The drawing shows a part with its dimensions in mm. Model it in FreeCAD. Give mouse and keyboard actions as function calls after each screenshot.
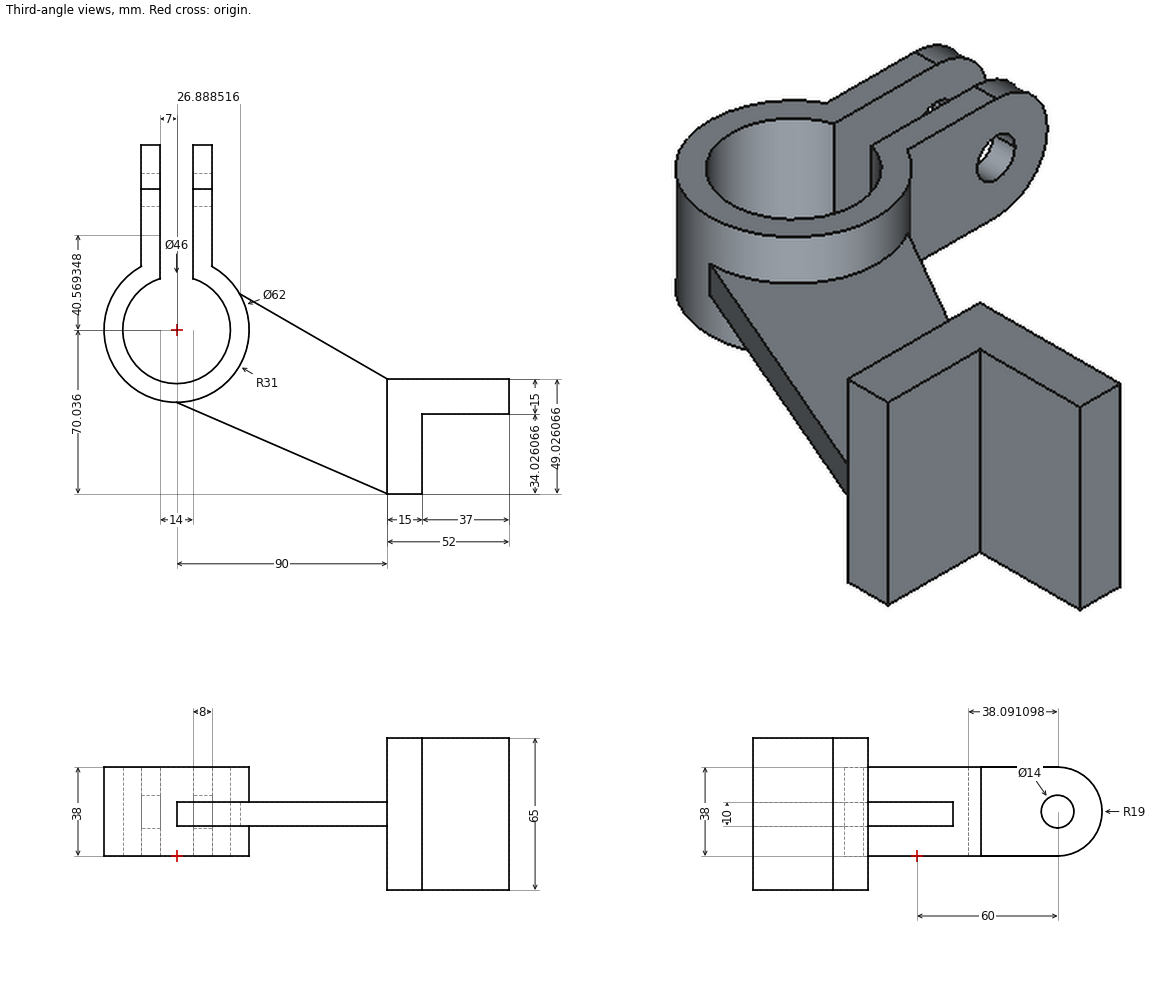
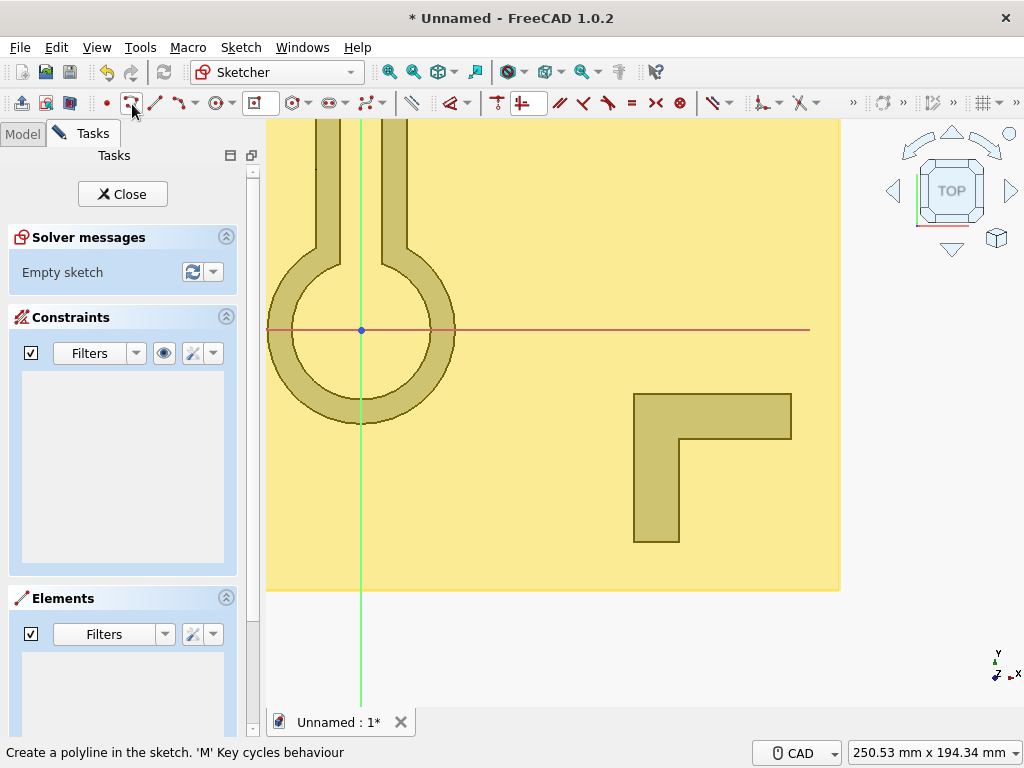
click(361, 424)
click(634, 542)
click(679, 542)
click(679, 439)
click(791, 439)
click(791, 394)
click(634, 394)
click(443, 283)
right_click(443, 283)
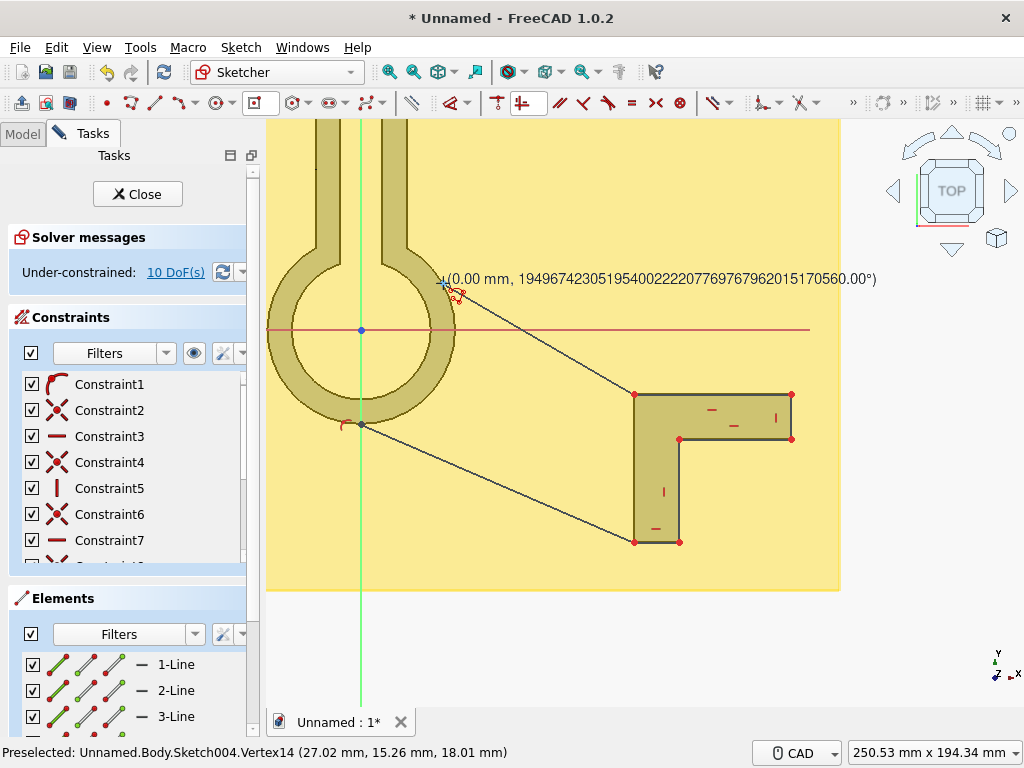
click(180, 104)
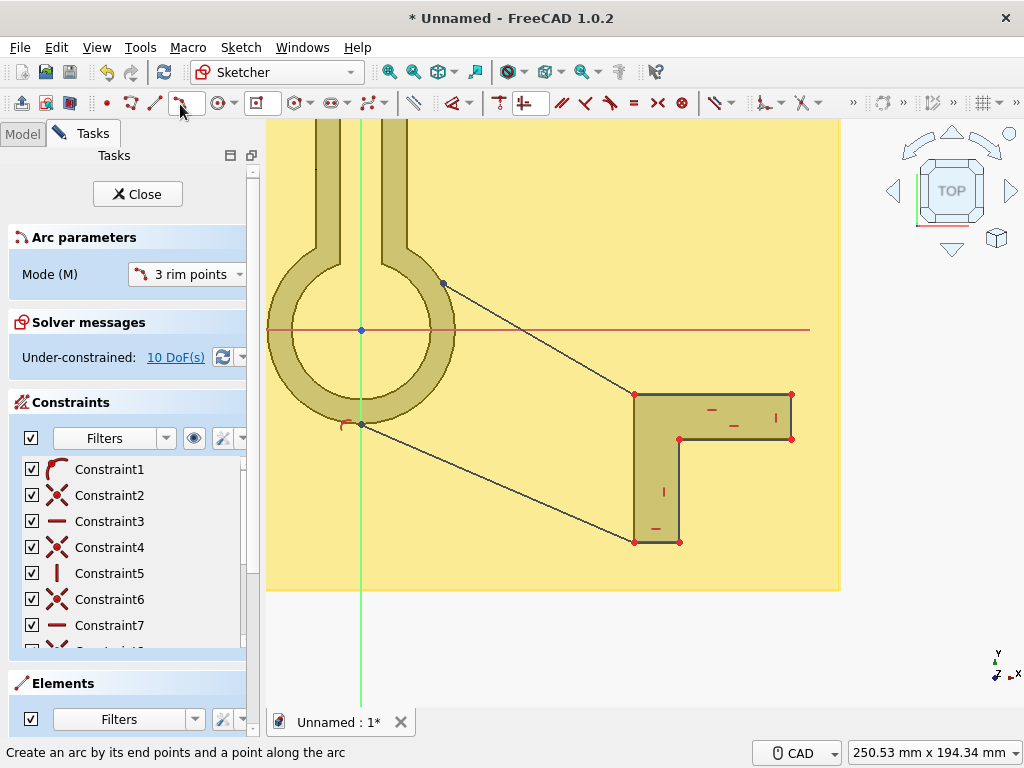
click(443, 284)
click(361, 425)
click(442, 377)
key(Escape)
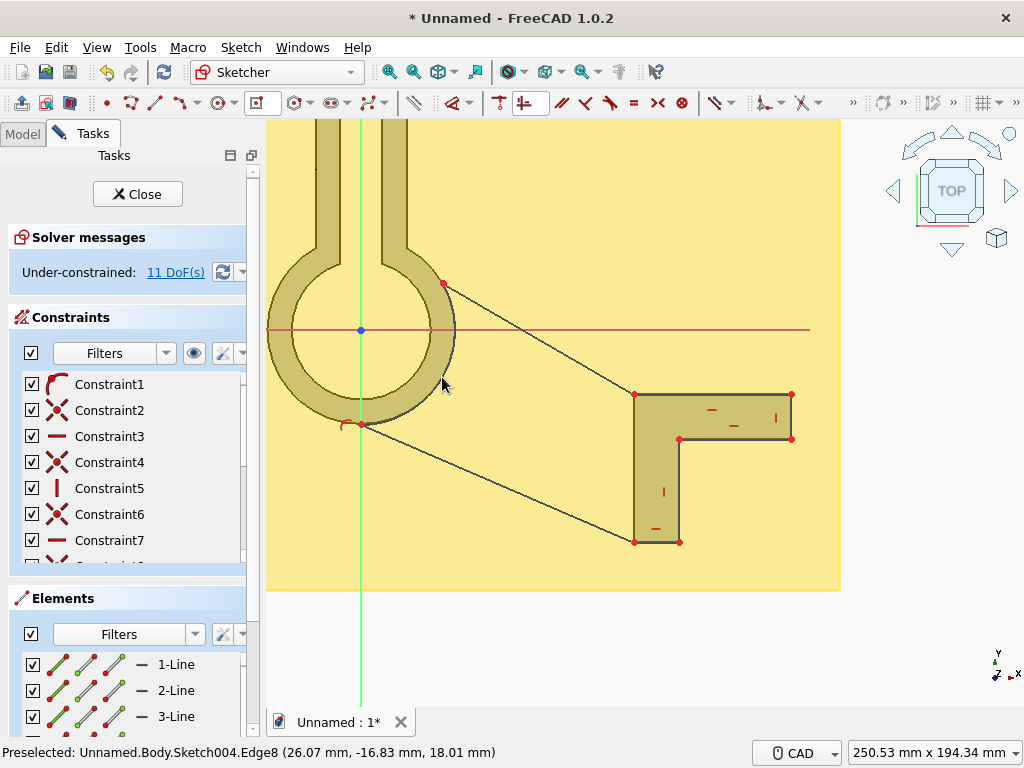
drag(350, 320, 371, 340)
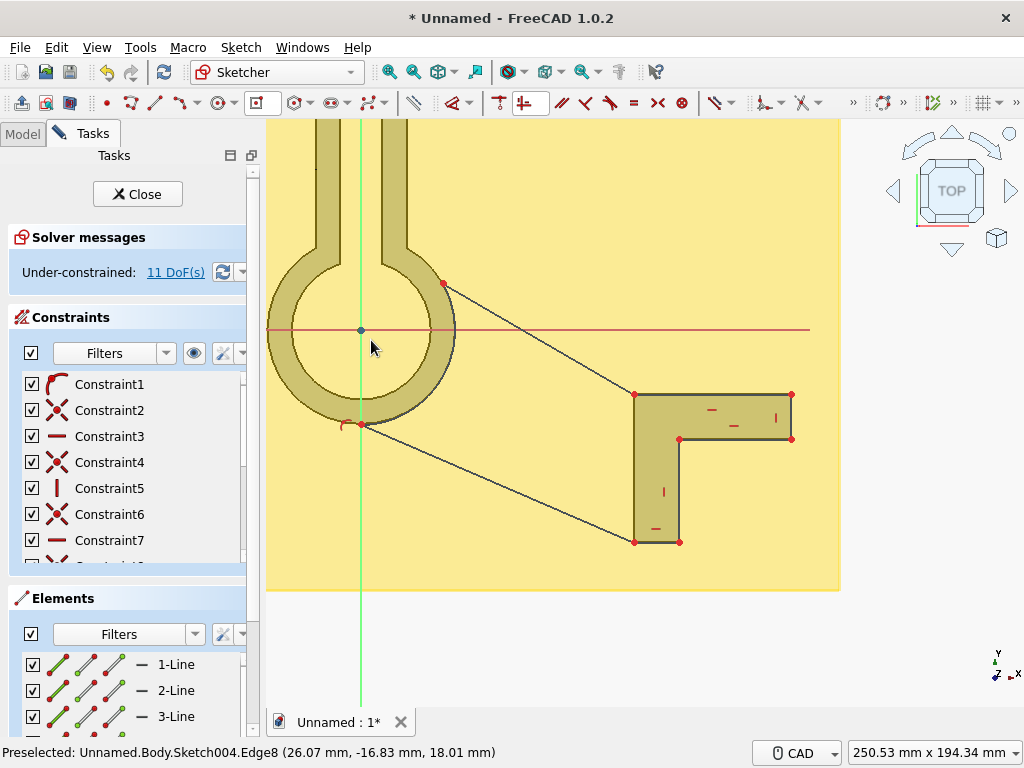
click(500, 104)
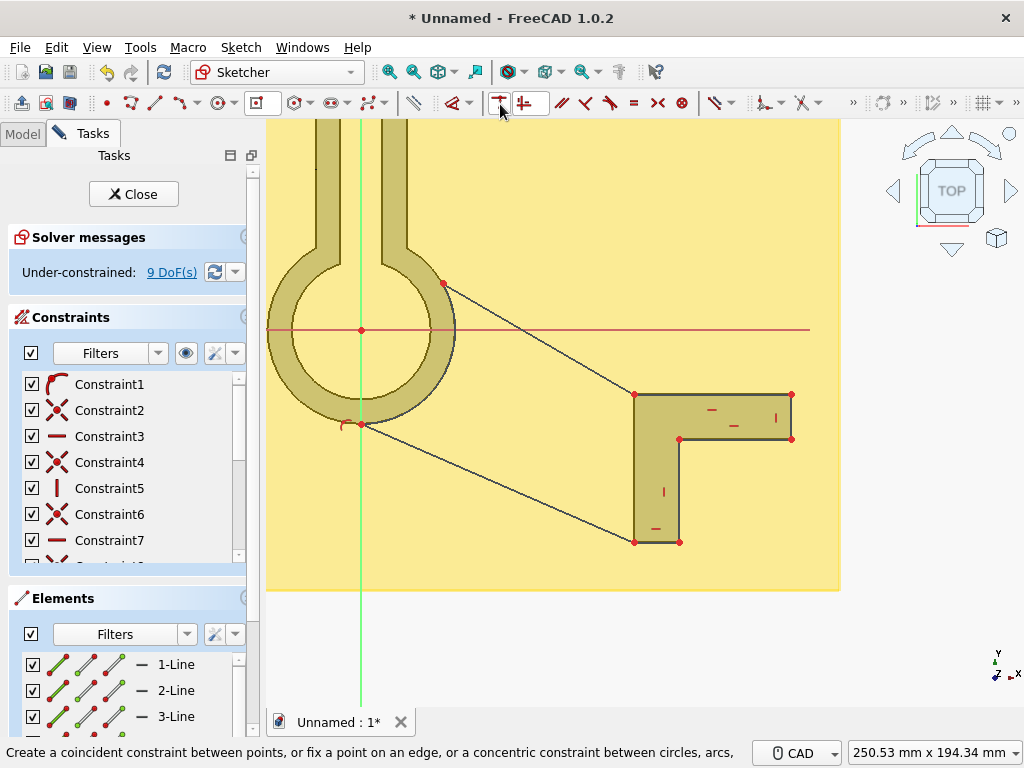
key(d)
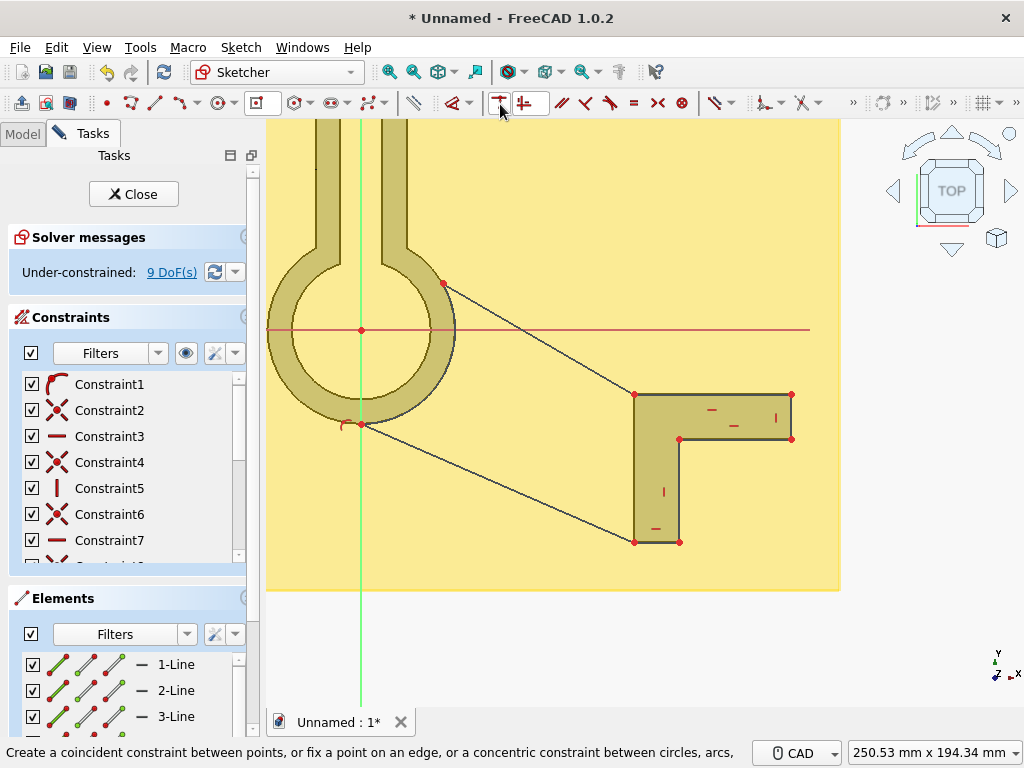
click(416, 406)
click(435, 432)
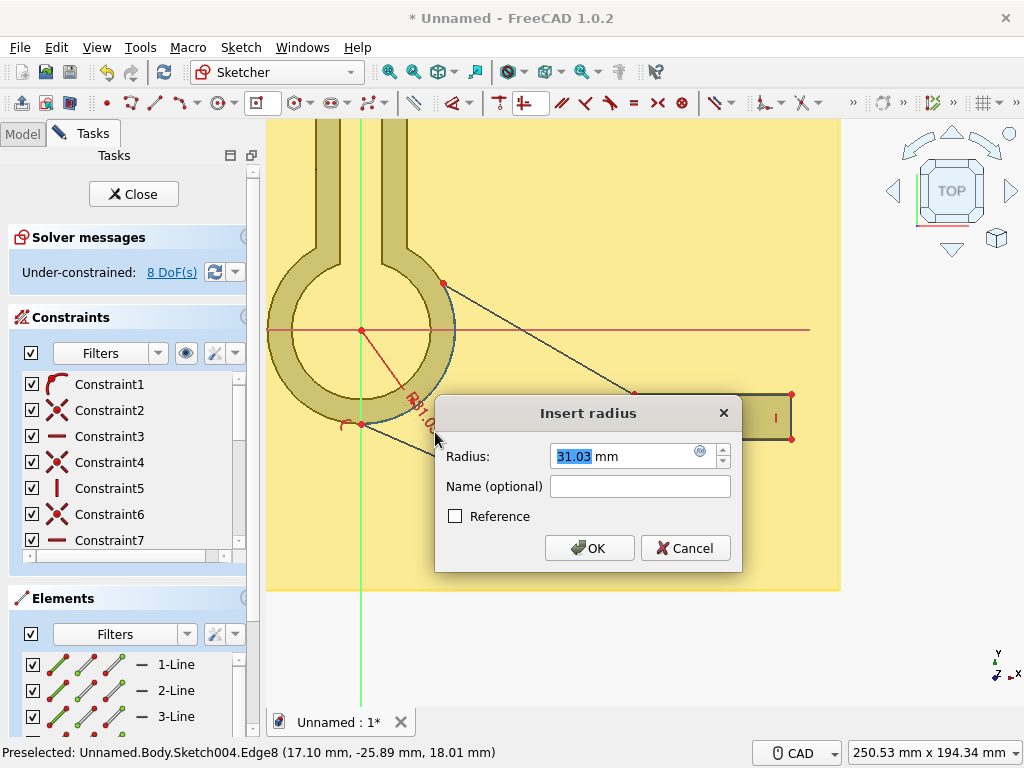
text(31)
key(Return)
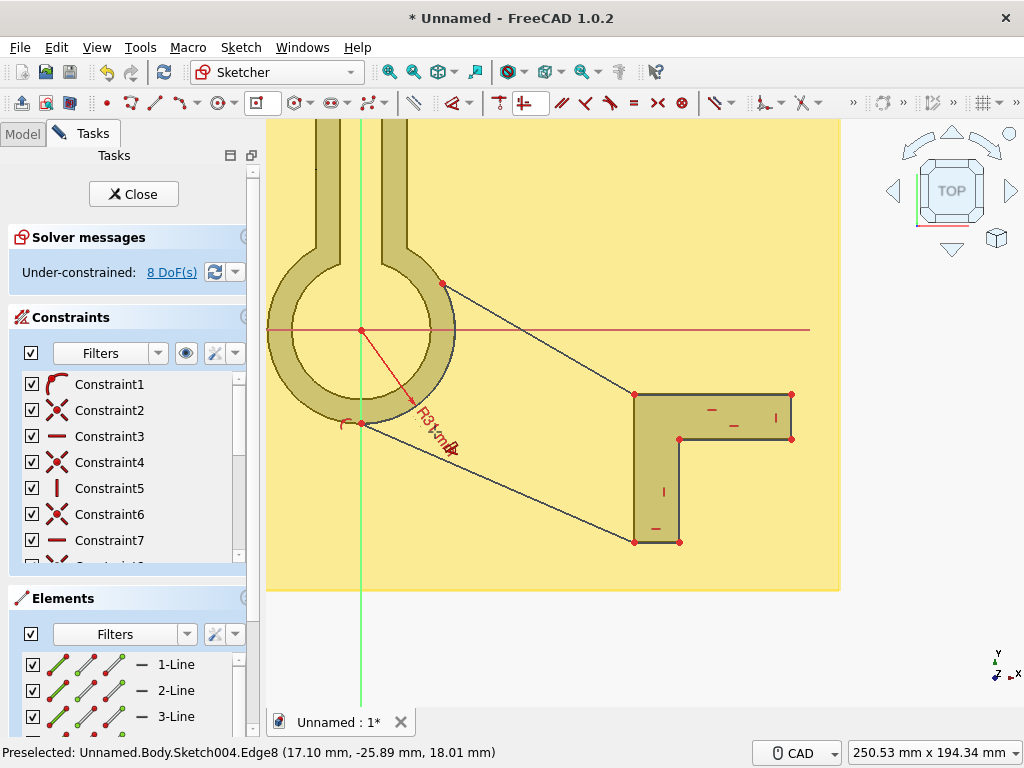
click(647, 543)
click(656, 577)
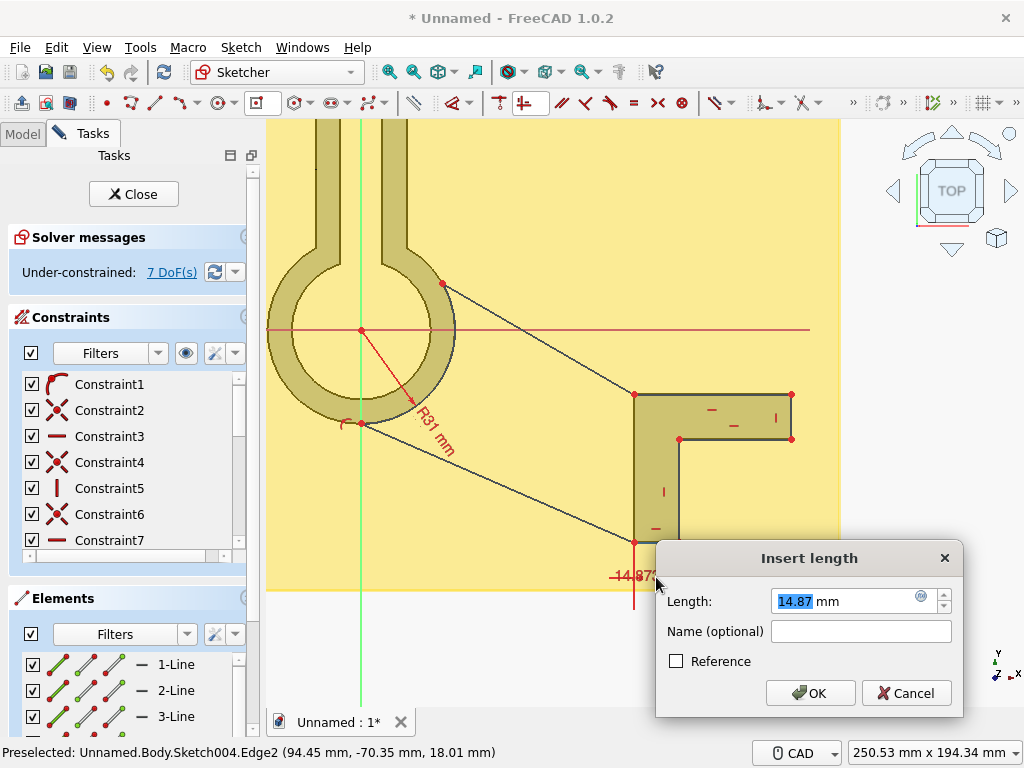
text(15)
key(Return)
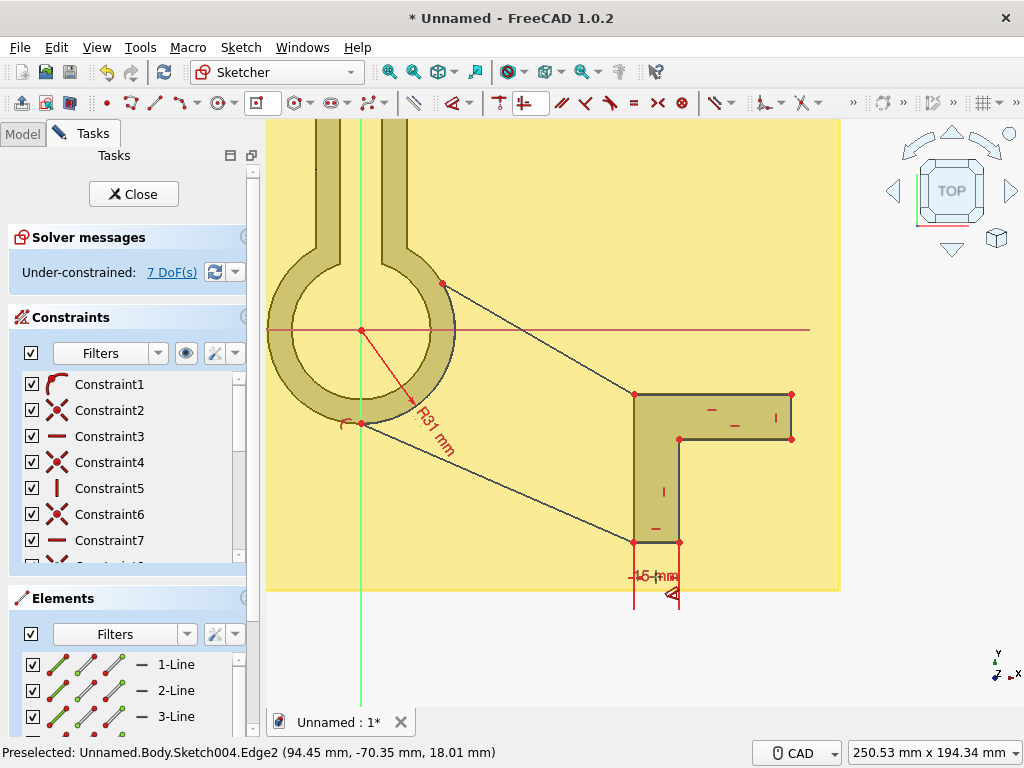
click(713, 440)
click(735, 474)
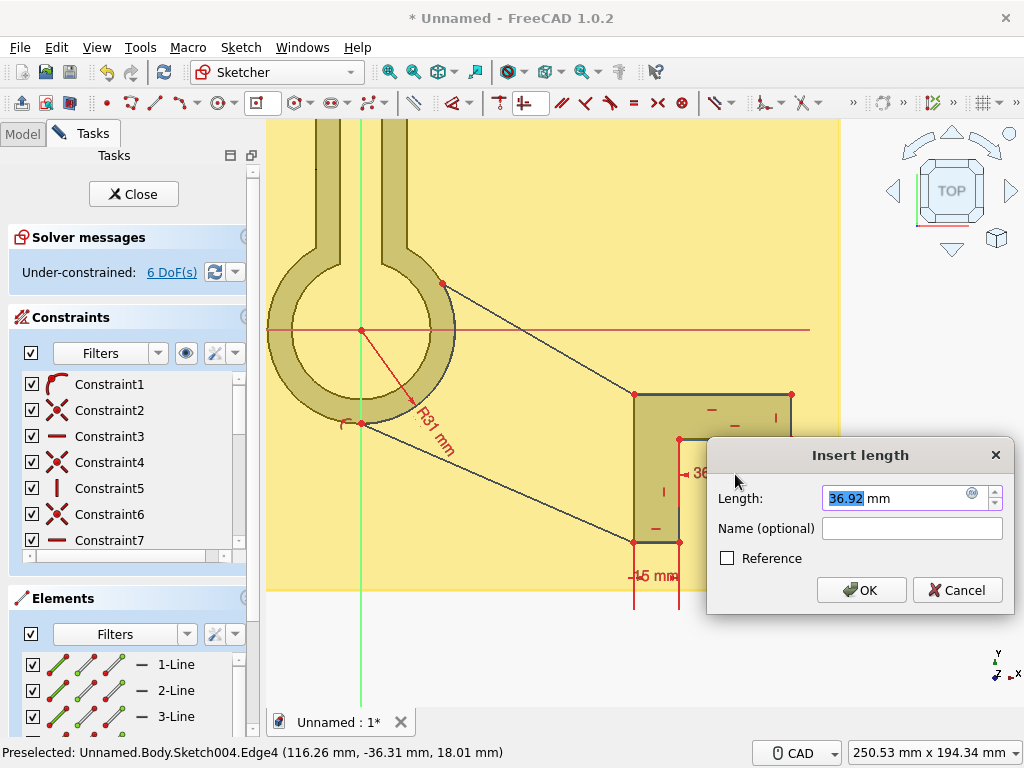
text(37)
key(Return)